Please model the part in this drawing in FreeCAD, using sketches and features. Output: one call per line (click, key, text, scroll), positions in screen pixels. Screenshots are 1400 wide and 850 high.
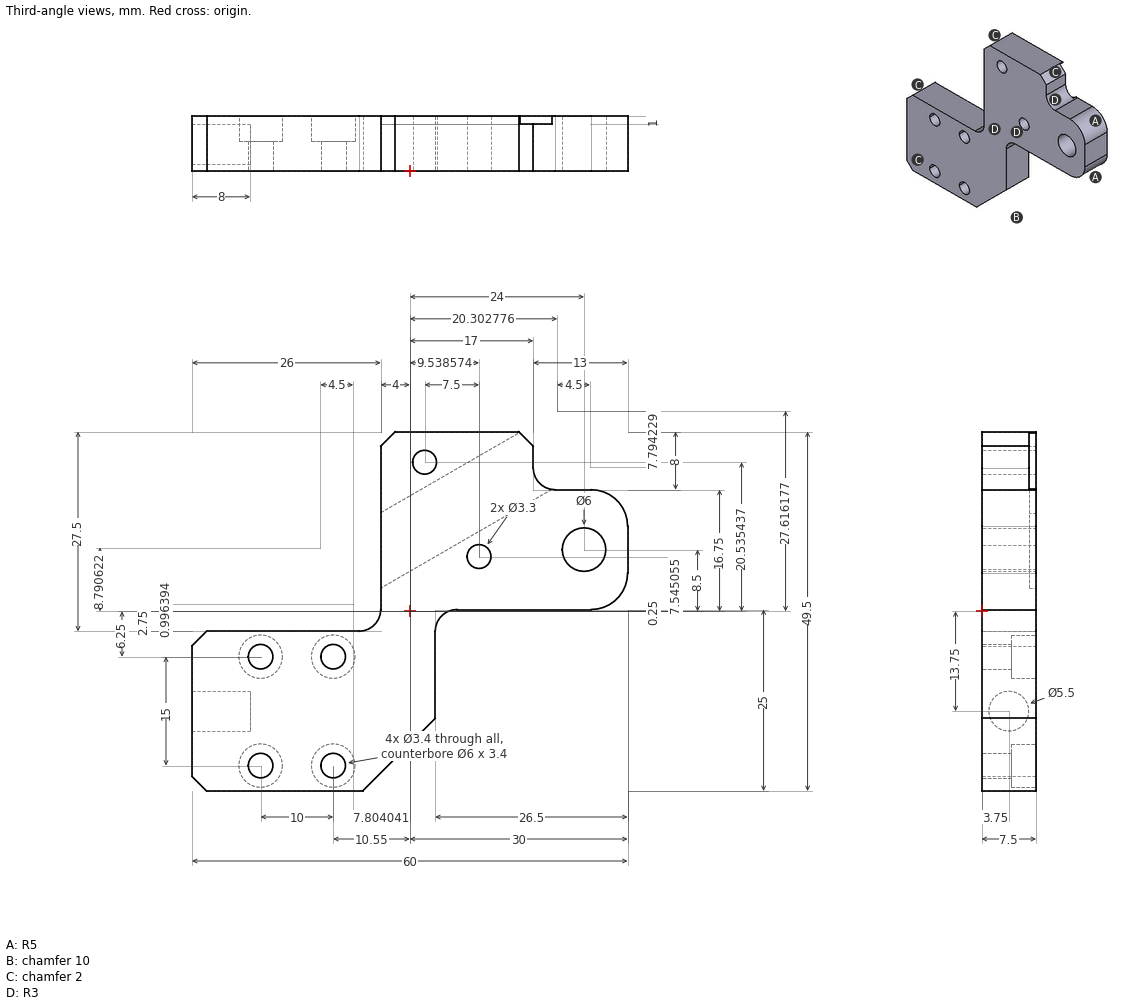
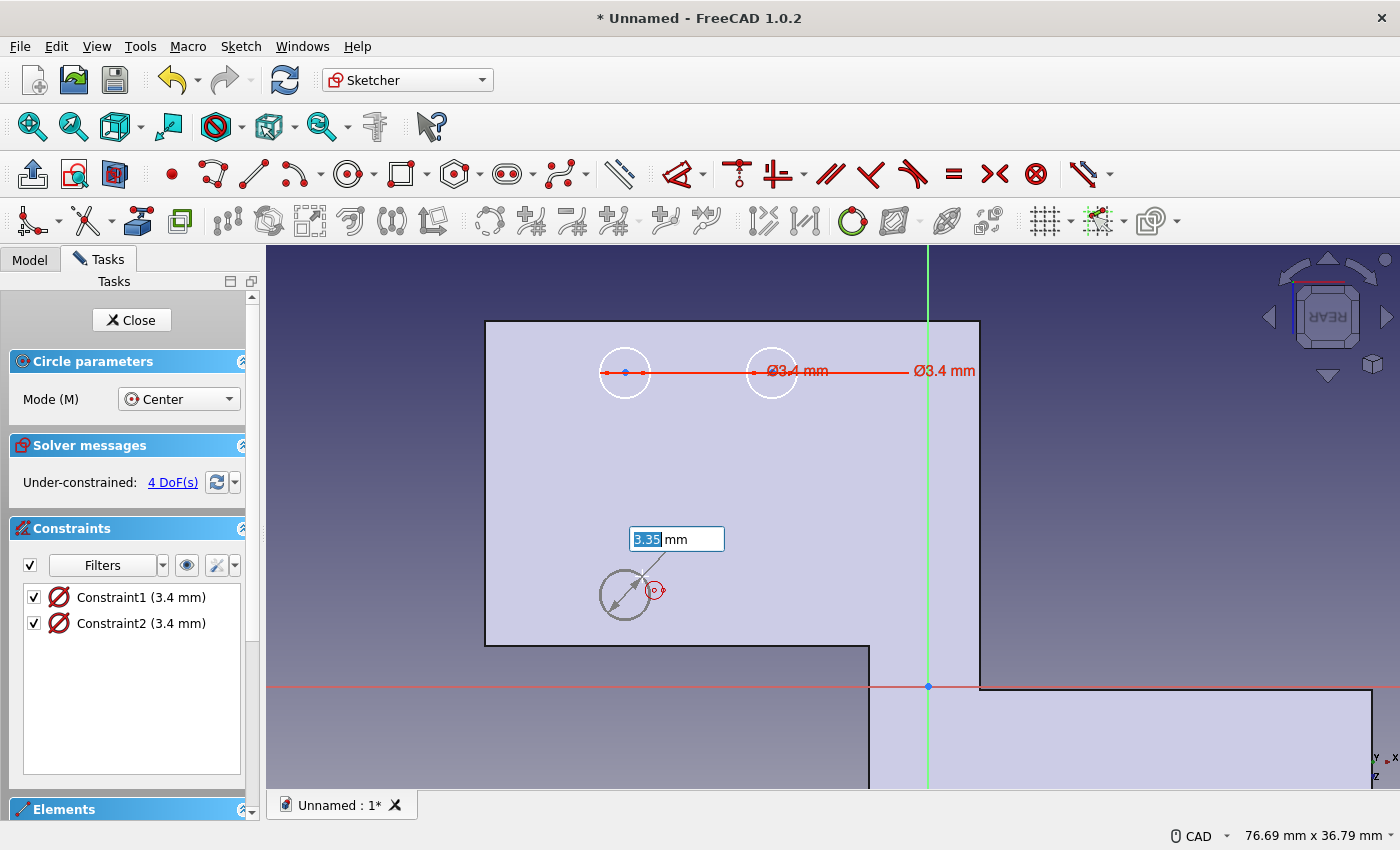
text(3.4)
key(Return)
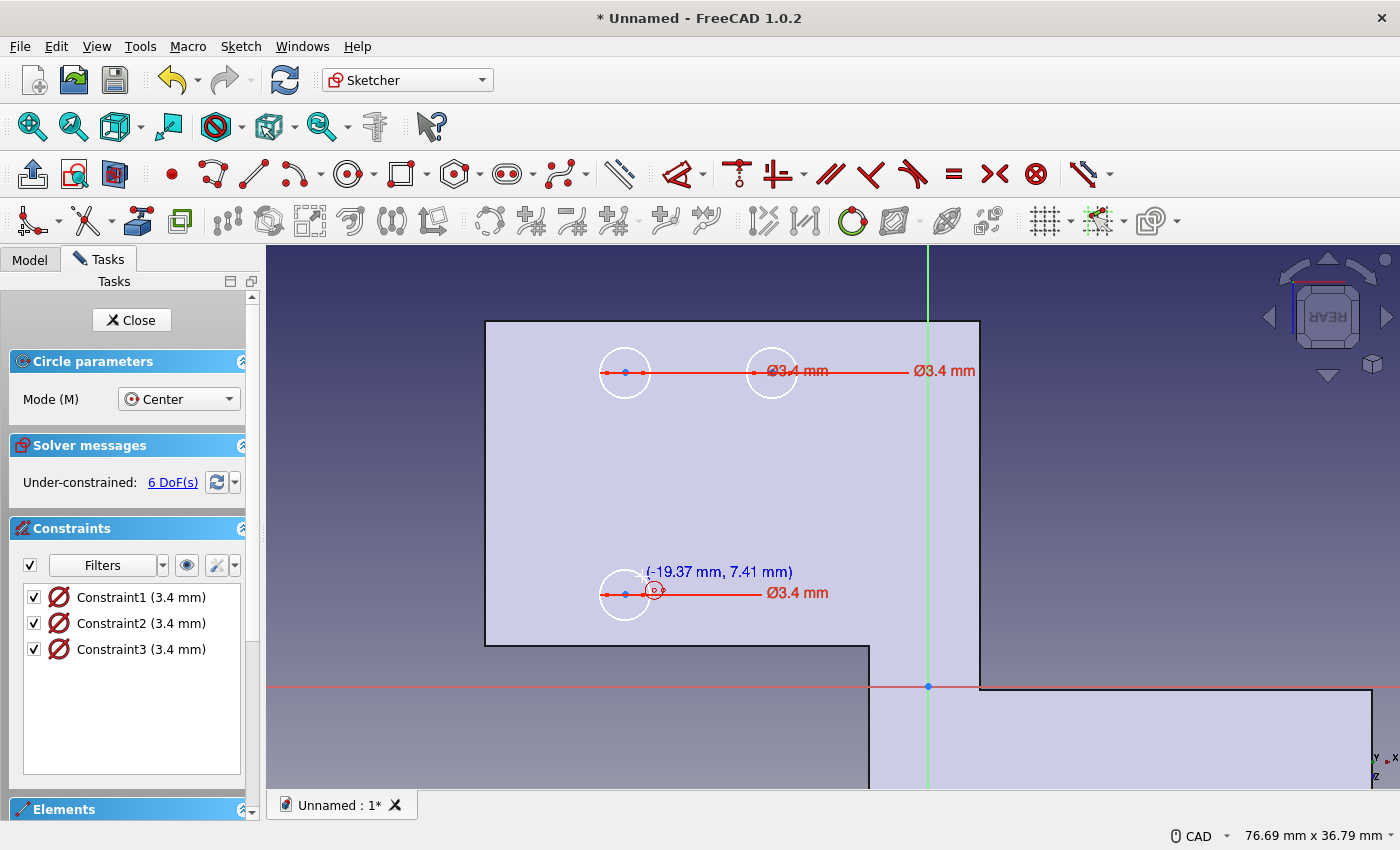
click(772, 594)
move(790, 576)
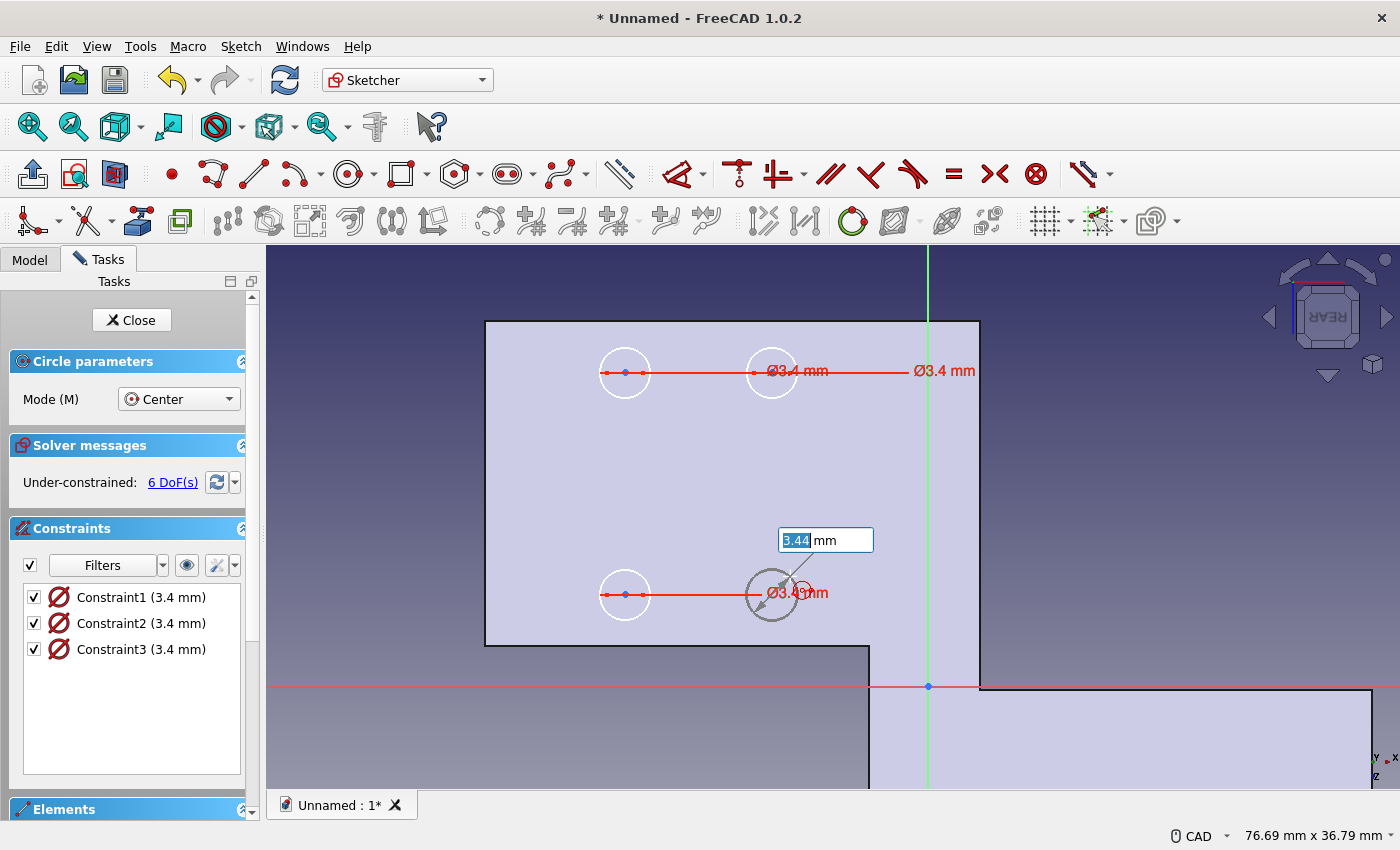
text(3.4)
key(Return)
key(Escape)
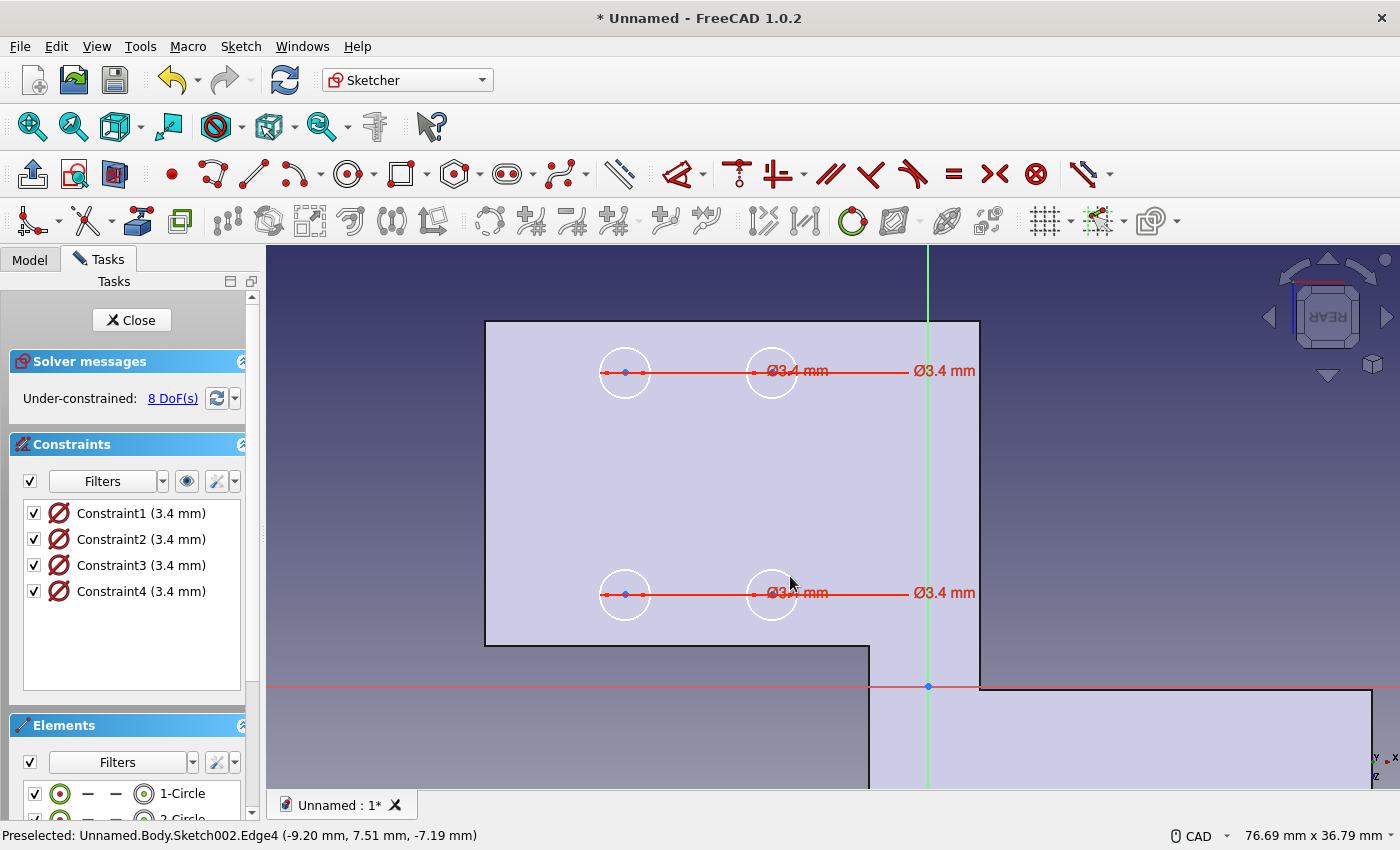
key(d)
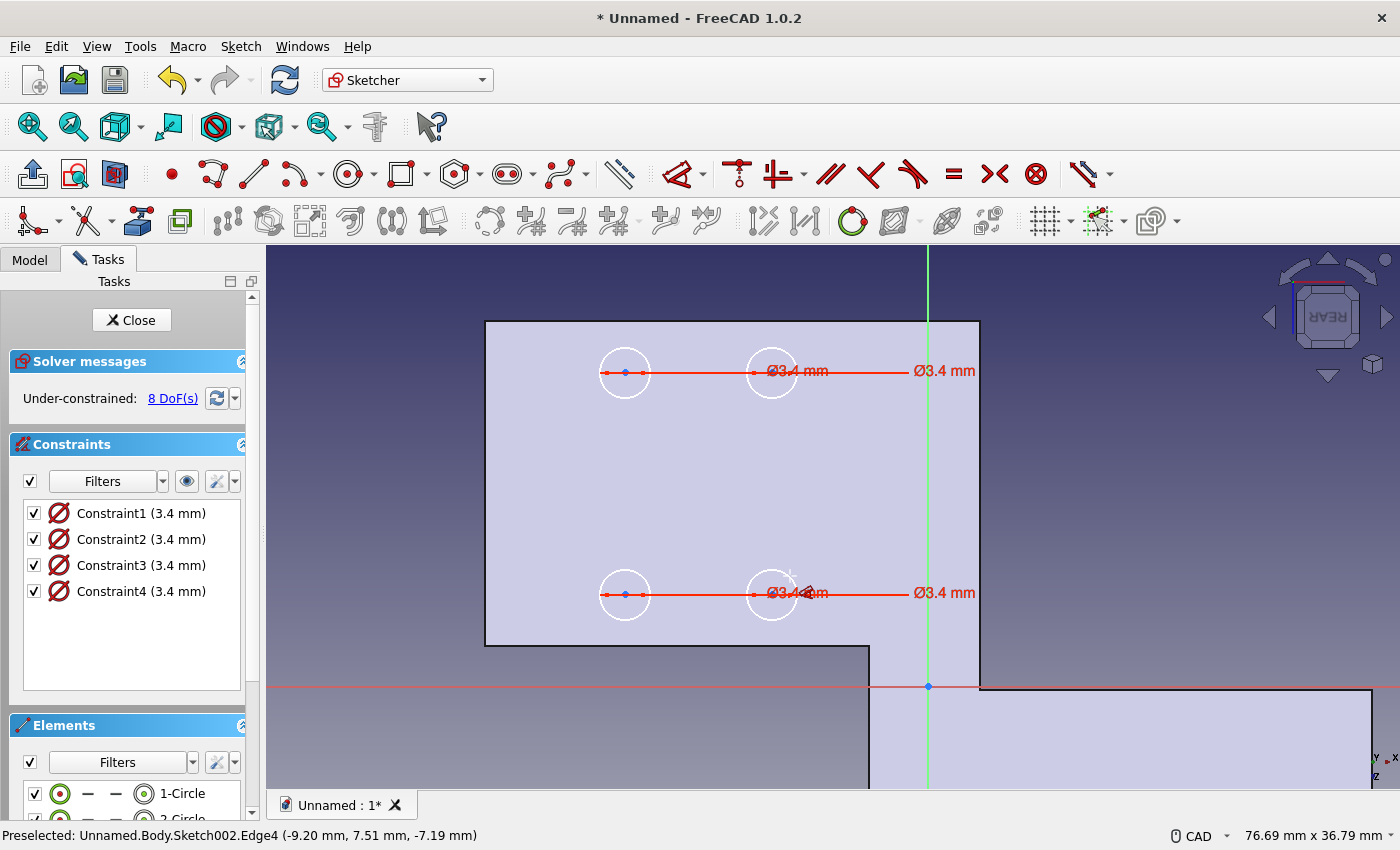
click(772, 373)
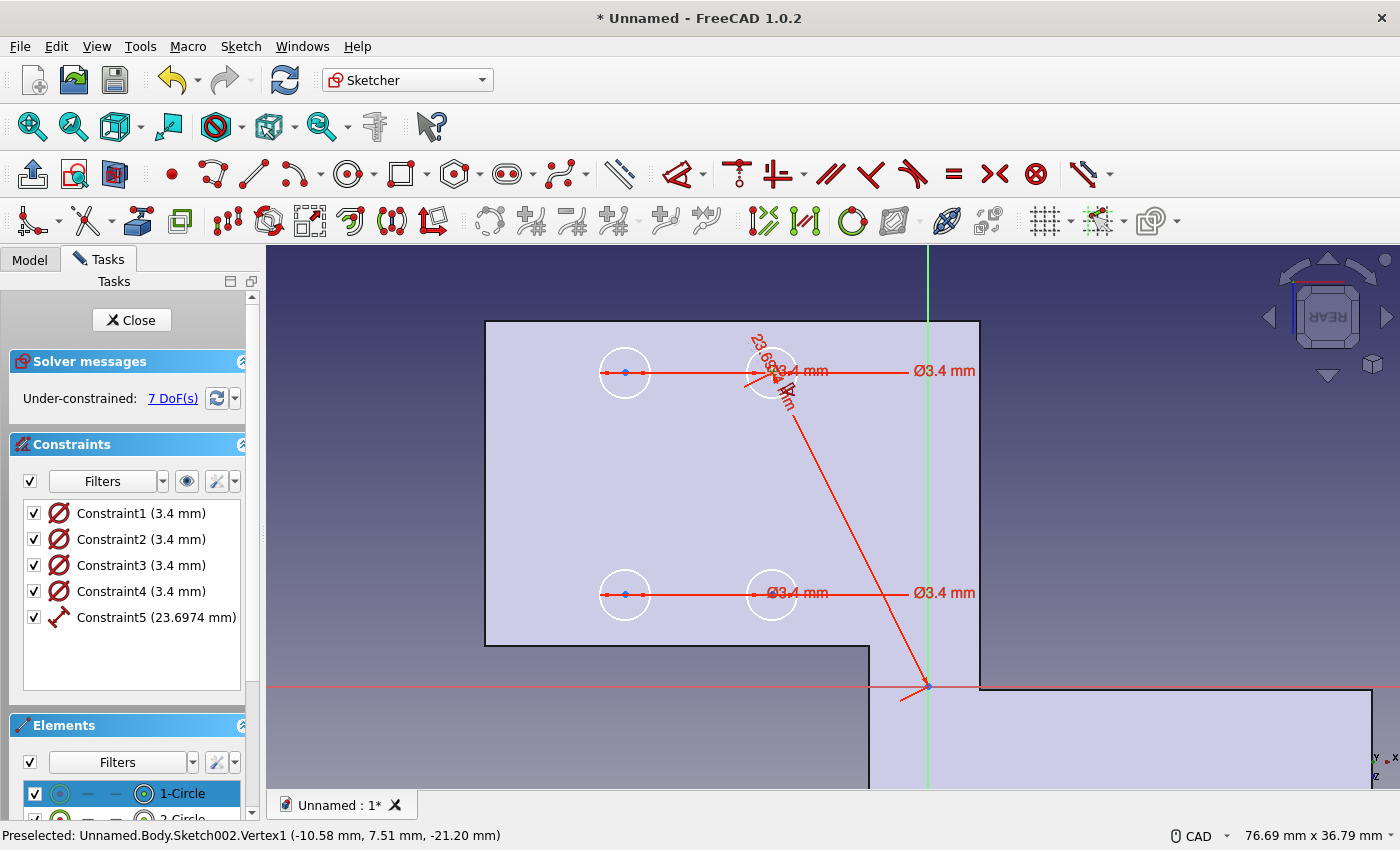
click(625, 373)
click(699, 339)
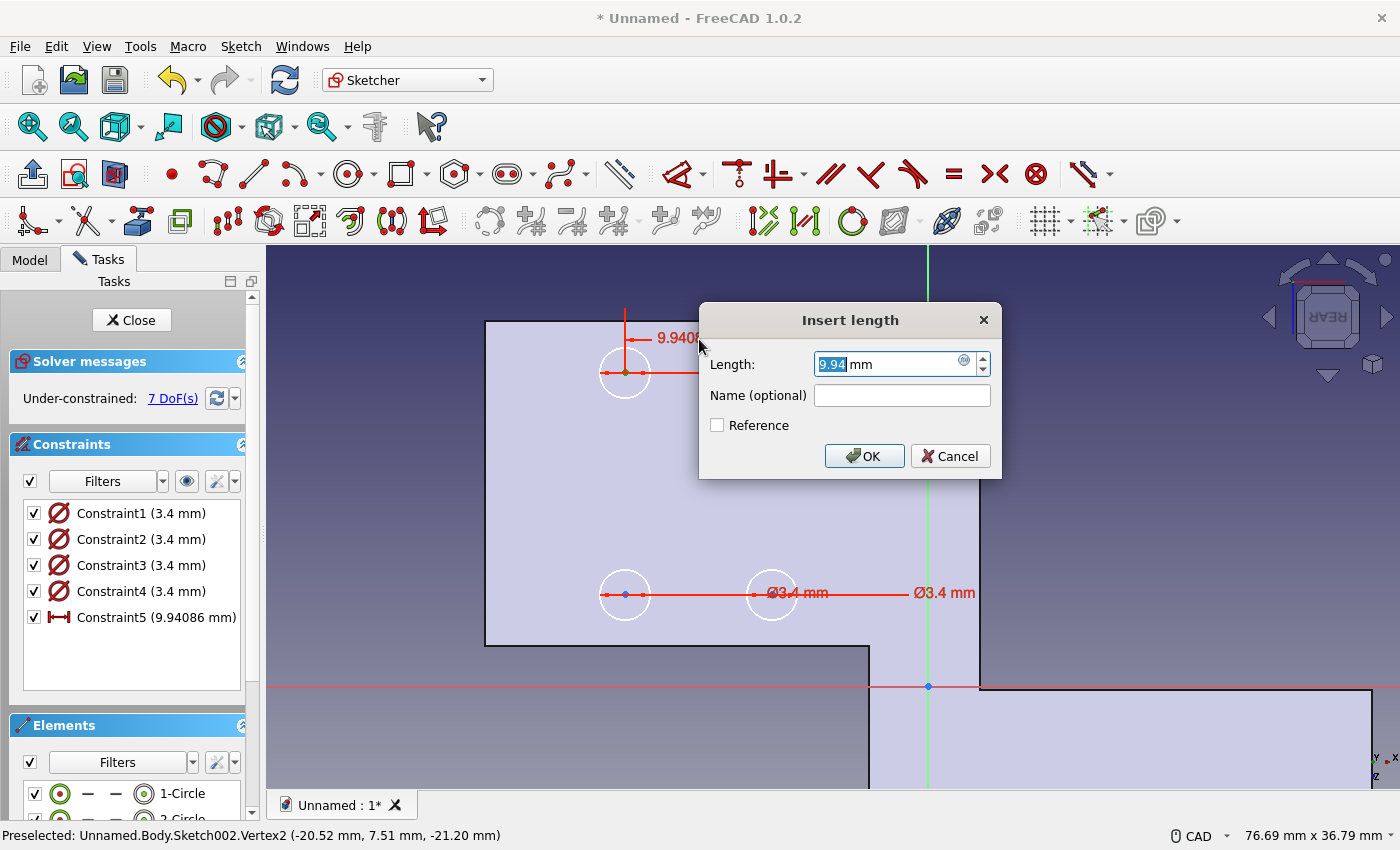
text(10)
key(Return)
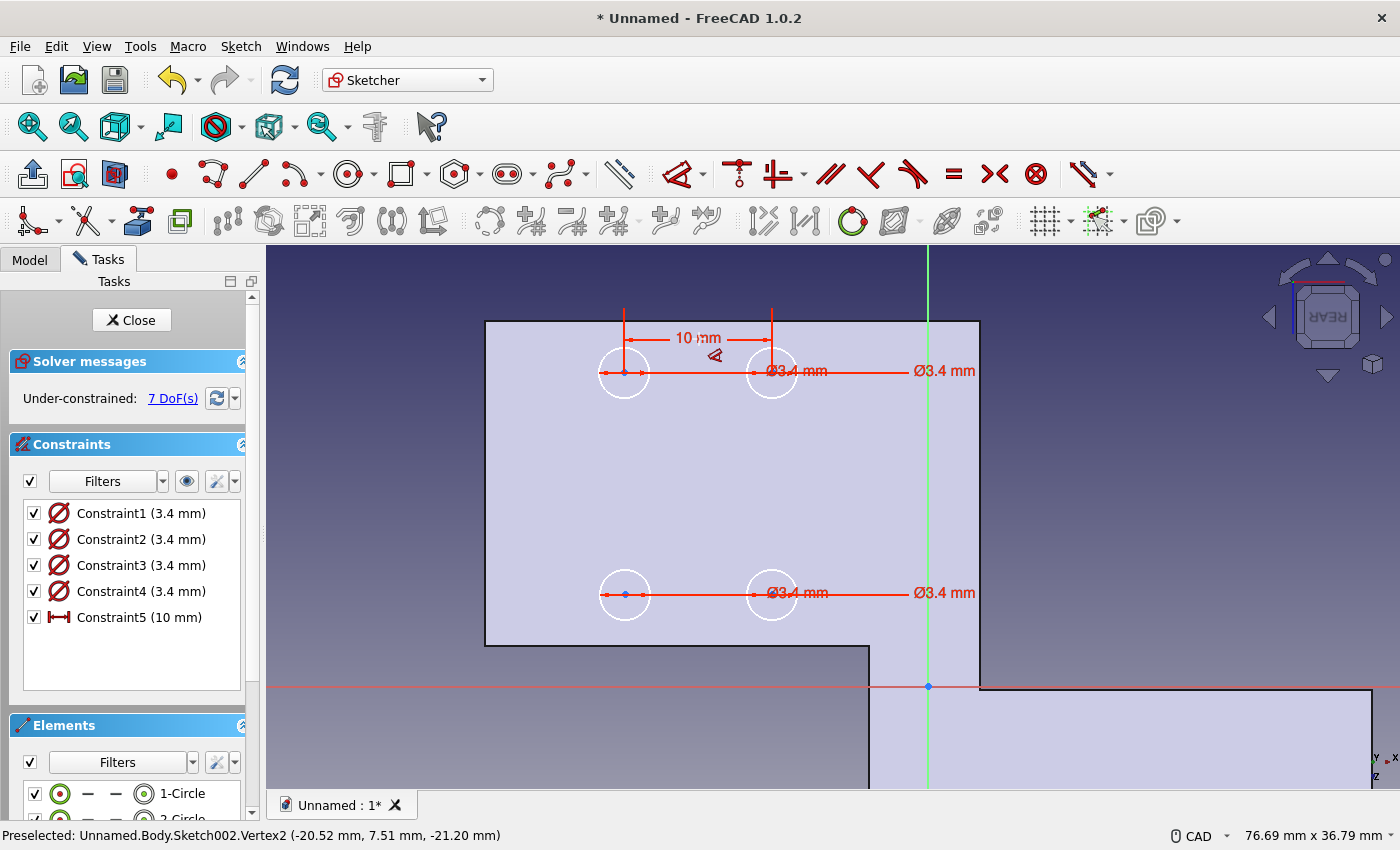
click(772, 373)